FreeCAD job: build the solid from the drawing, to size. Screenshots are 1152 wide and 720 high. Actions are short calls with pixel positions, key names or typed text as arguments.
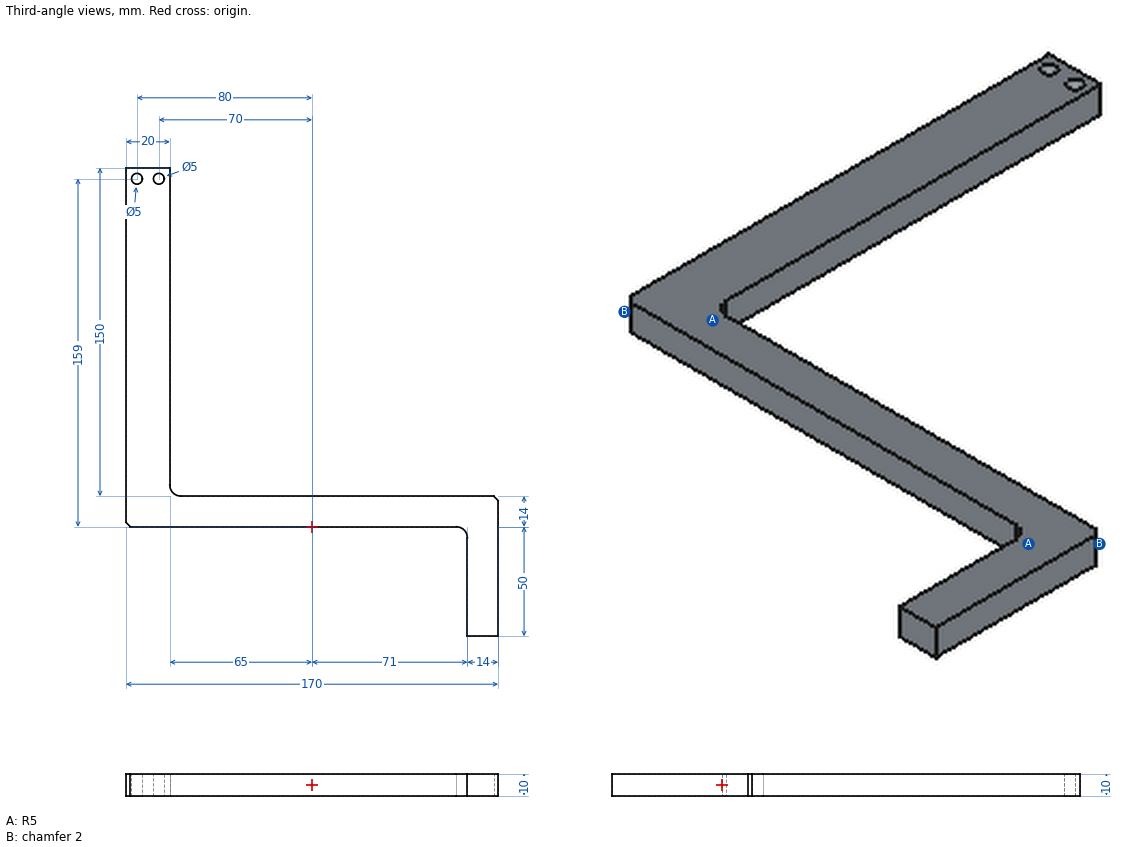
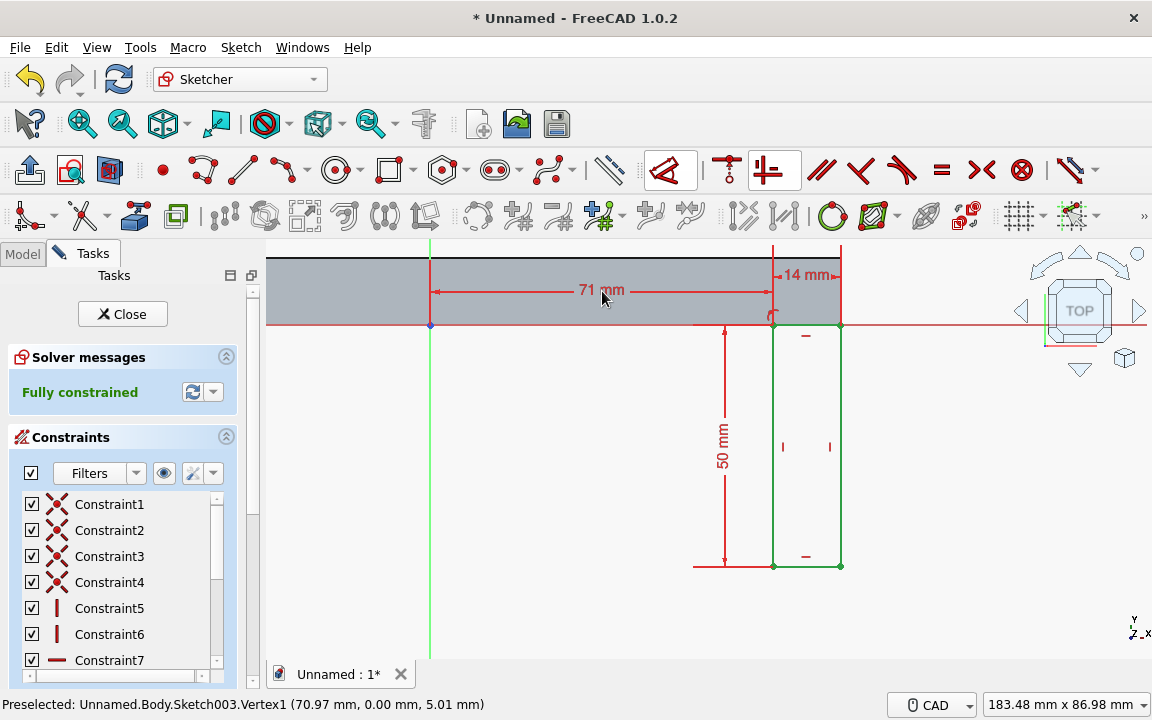
click(123, 314)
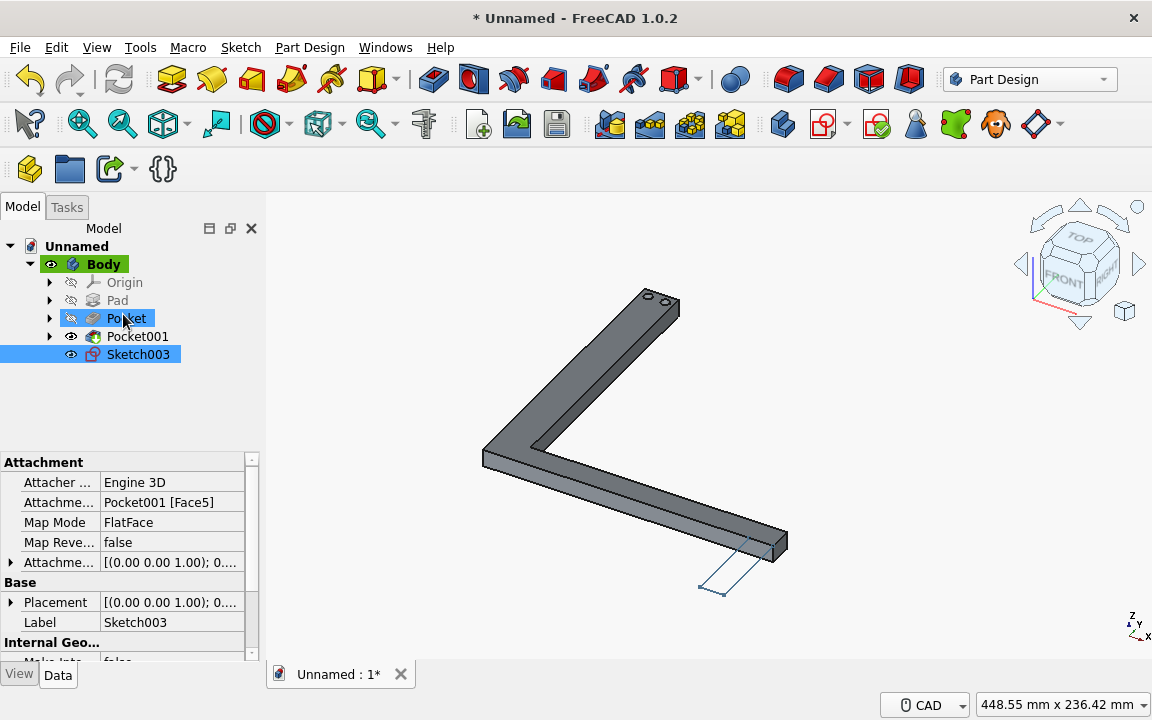
click(172, 80)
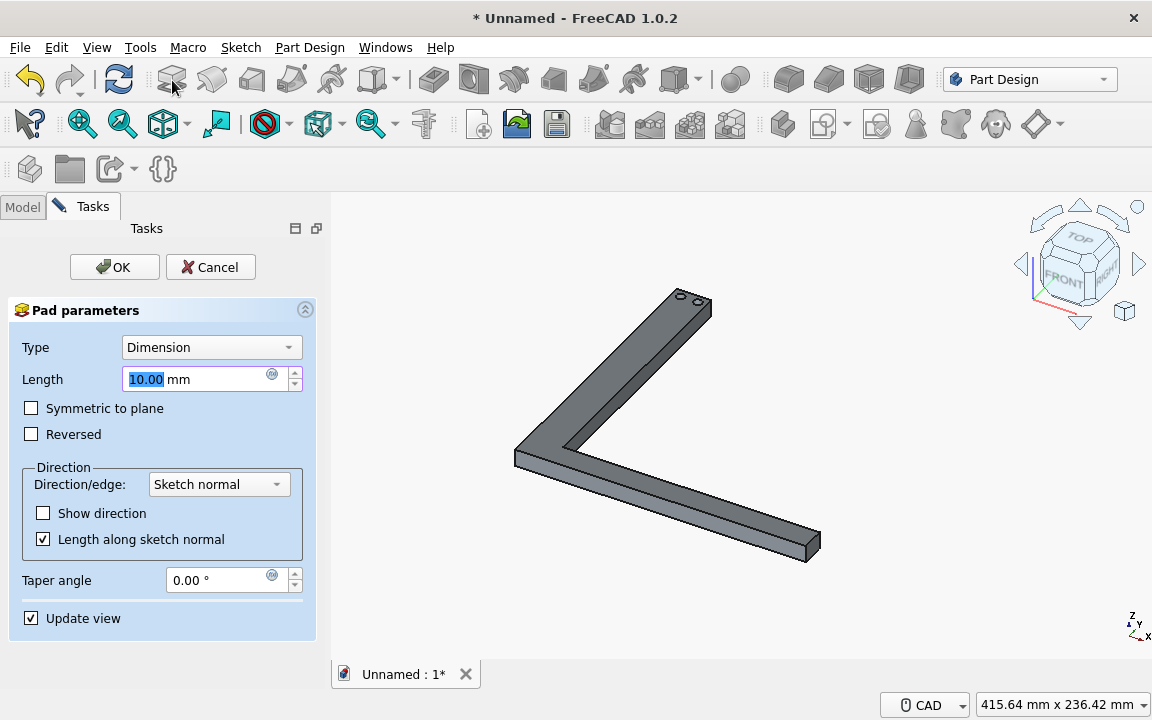
text(10)
key(Tab)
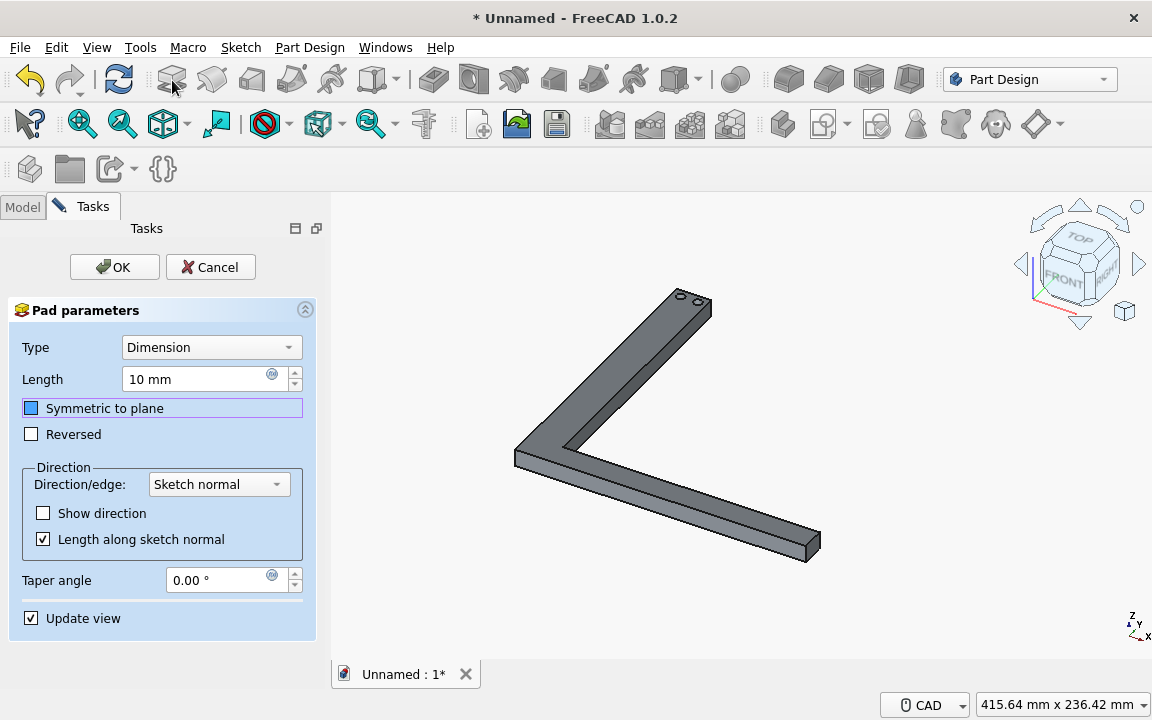
click(30, 434)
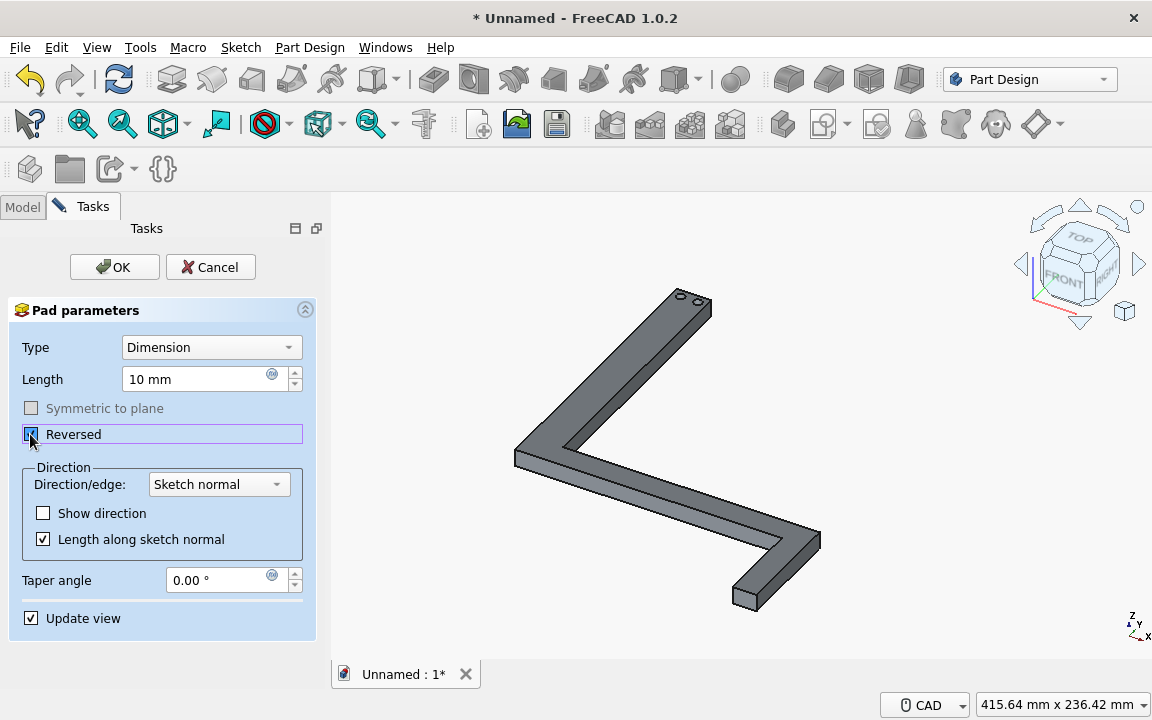
click(115, 267)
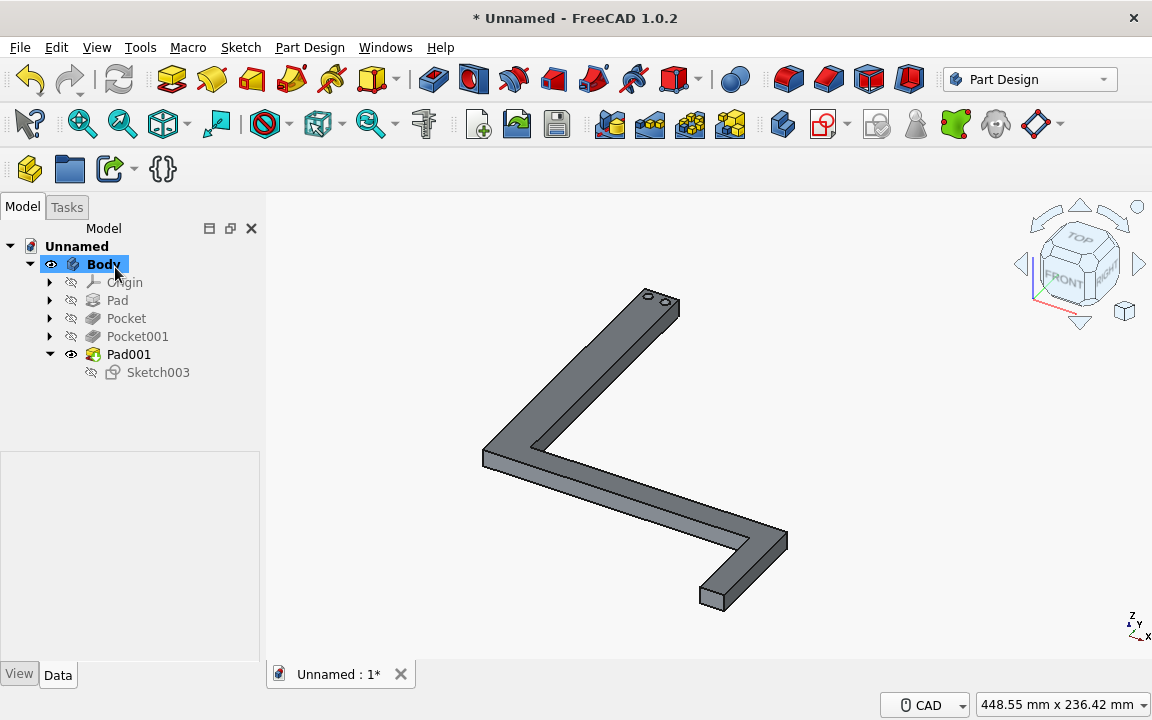
scroll(531, 454, up, 4)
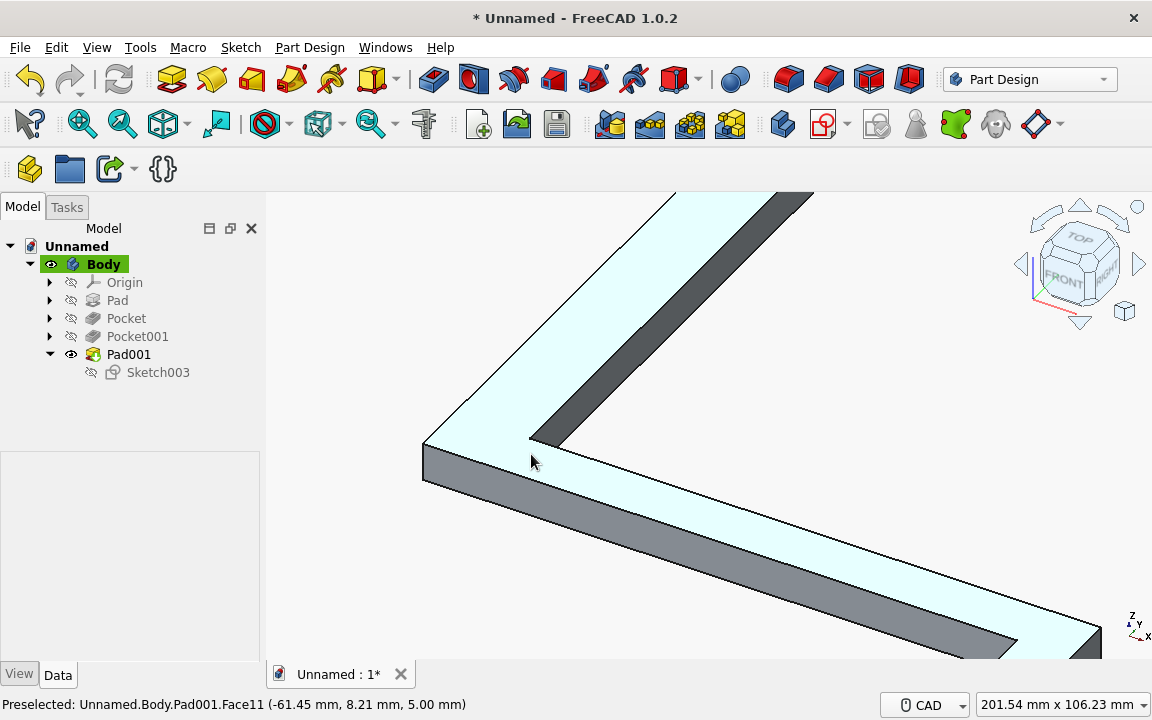
click(84, 124)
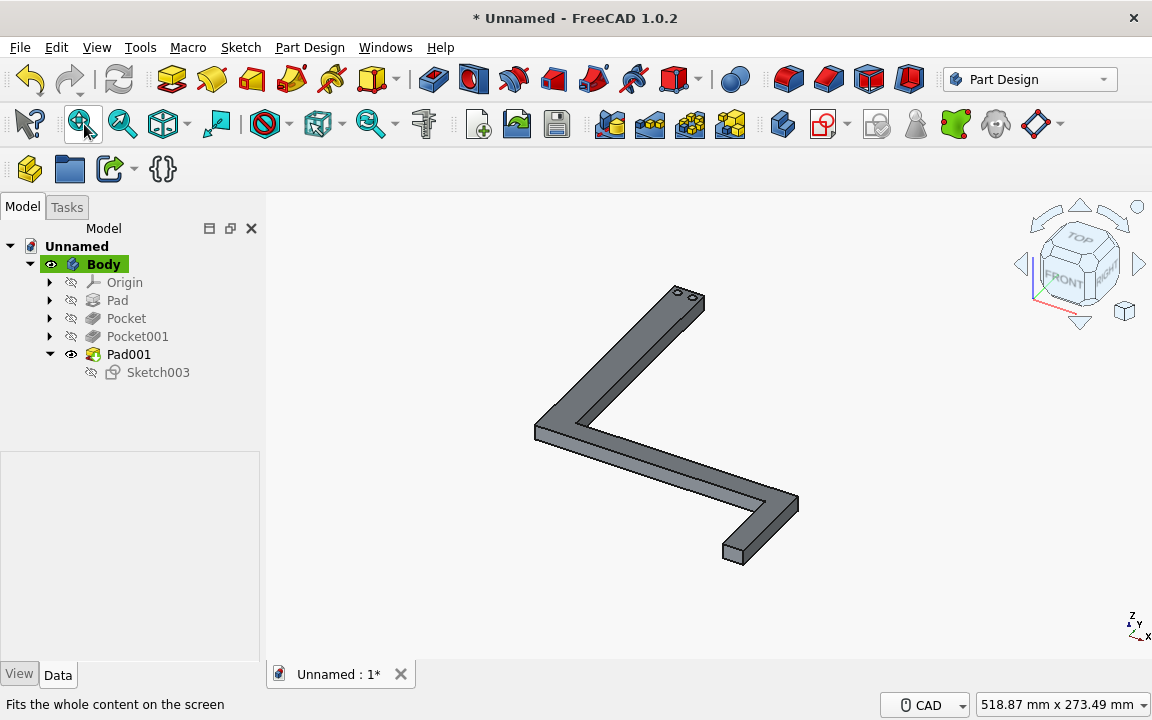
key(0)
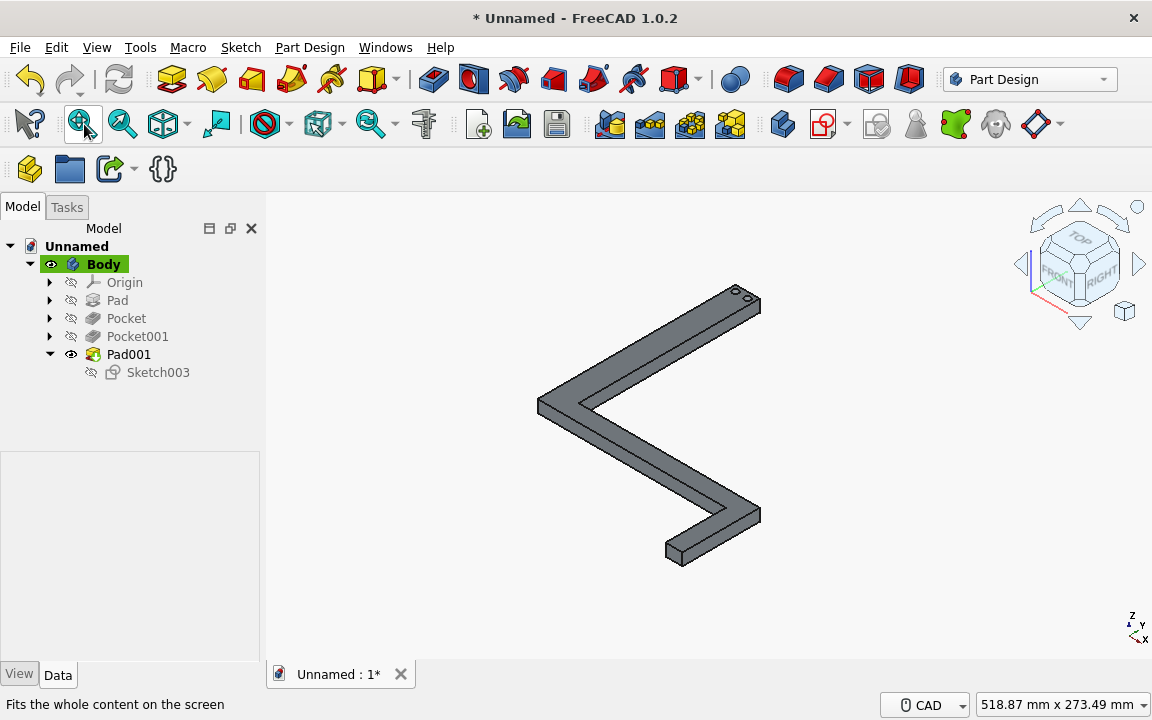
scroll(579, 409, up, 5)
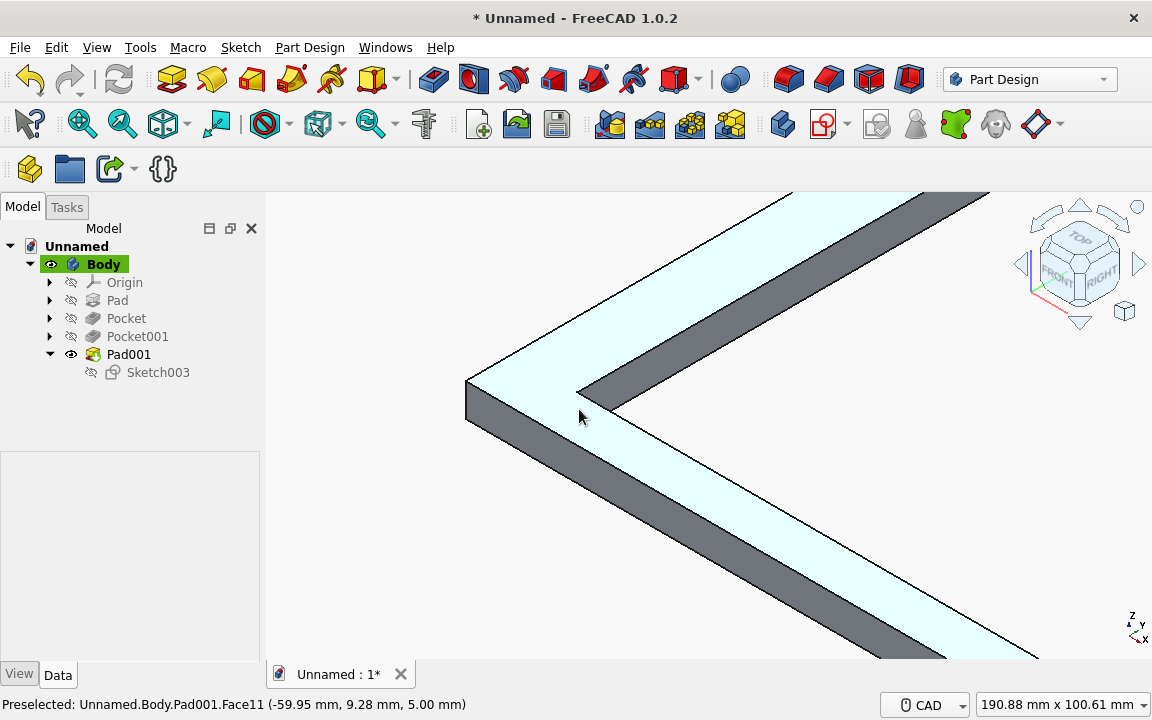
key(v)
key(f)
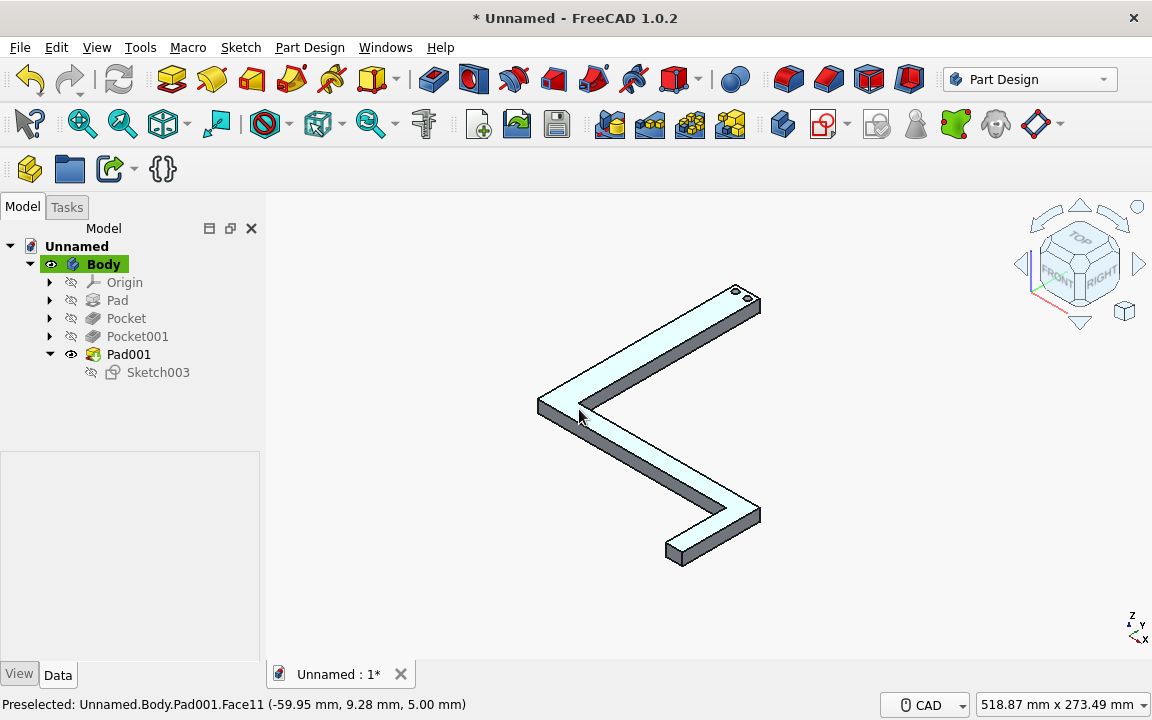
key(2)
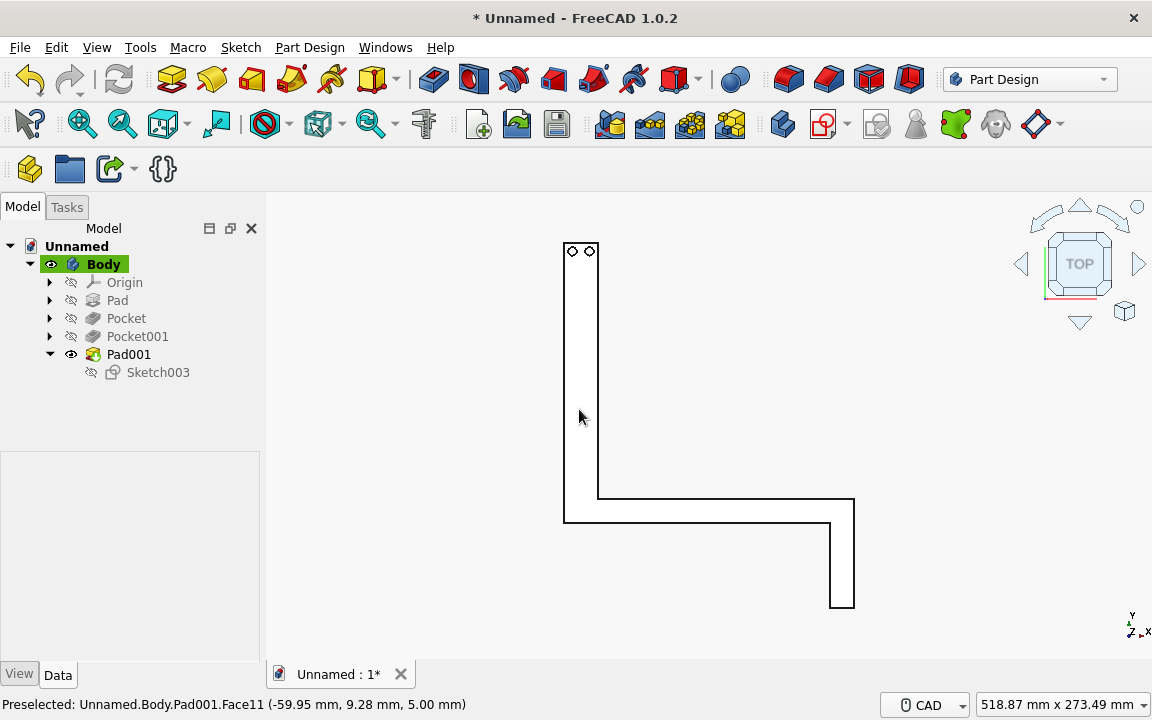
scroll(598, 498, up, 5)